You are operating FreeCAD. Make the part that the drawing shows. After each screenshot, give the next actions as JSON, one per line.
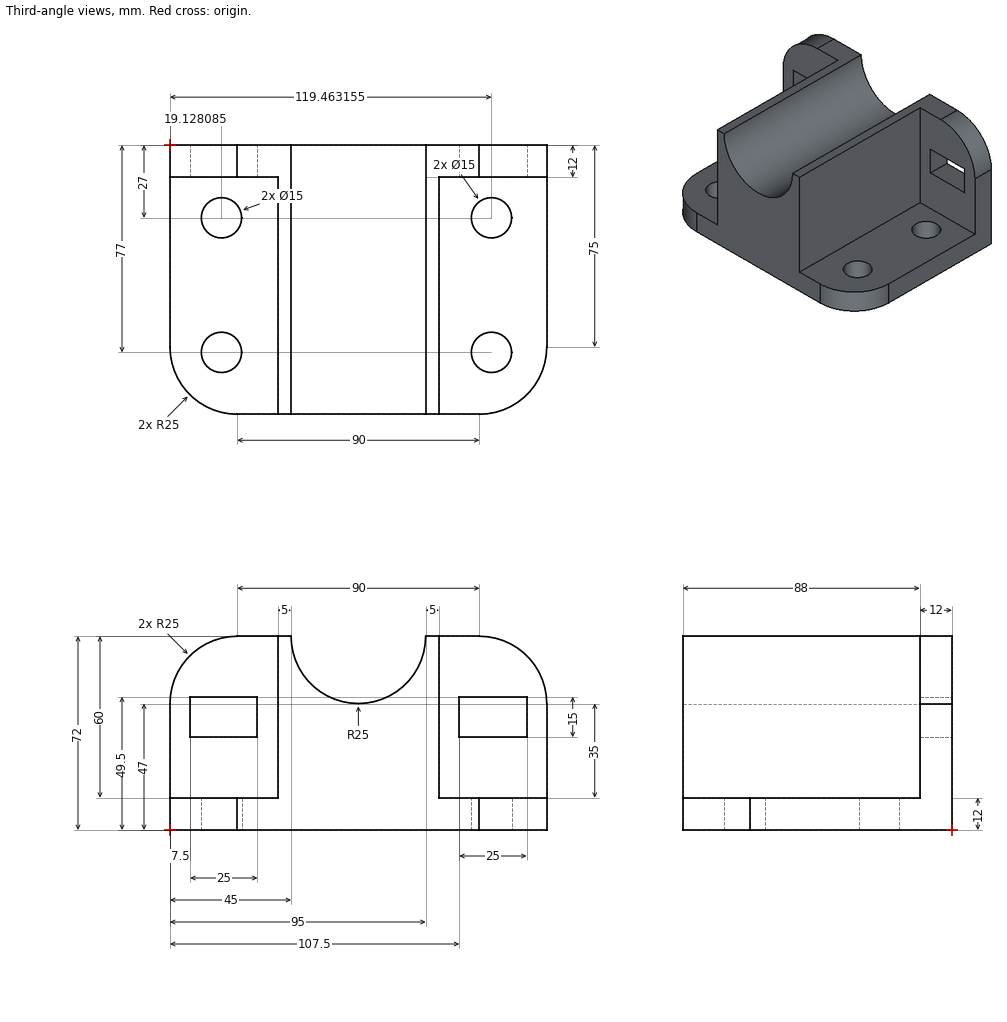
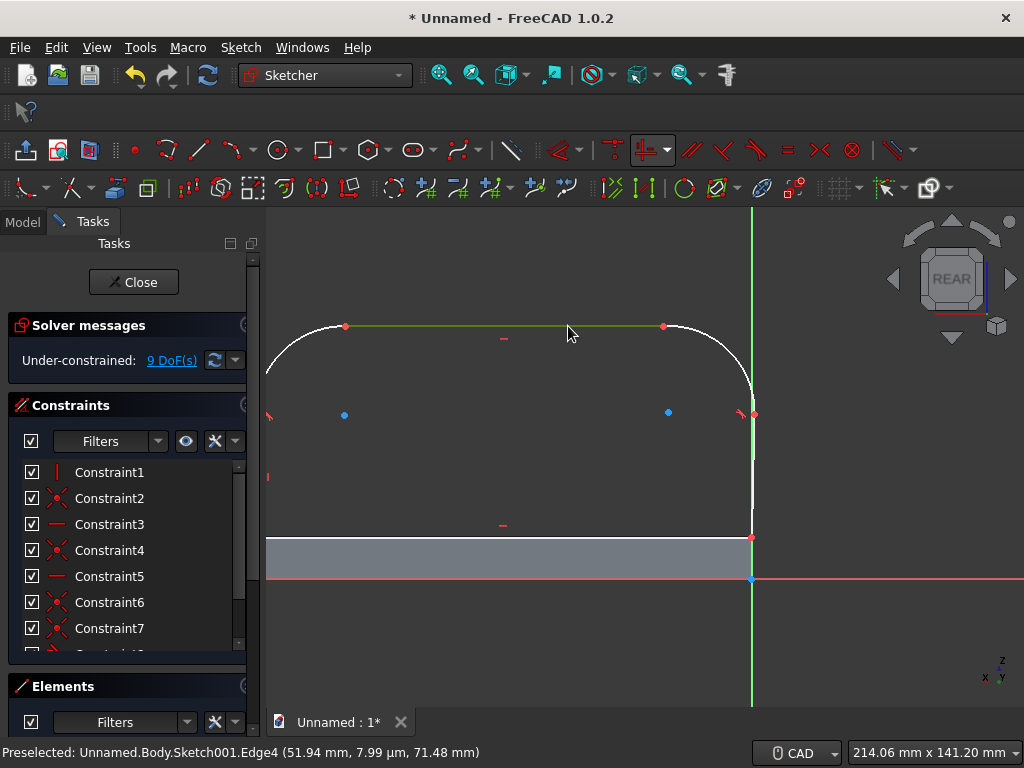
{"action": "left_click", "coordinate": [705, 334]}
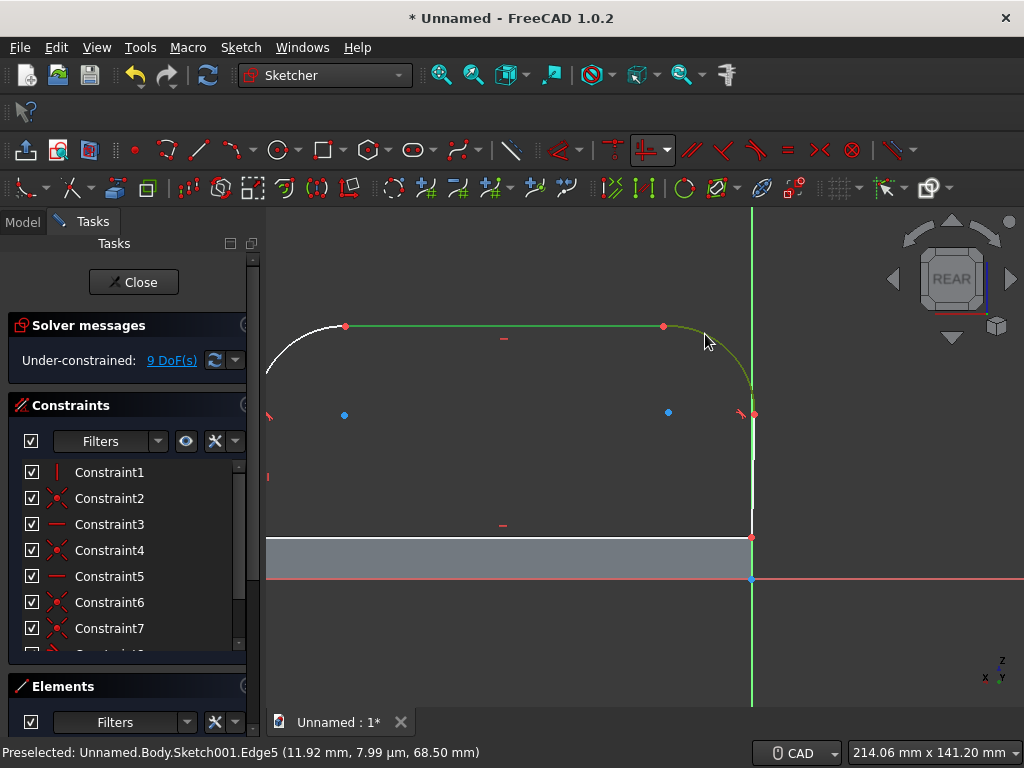
{"action": "key", "text": "t"}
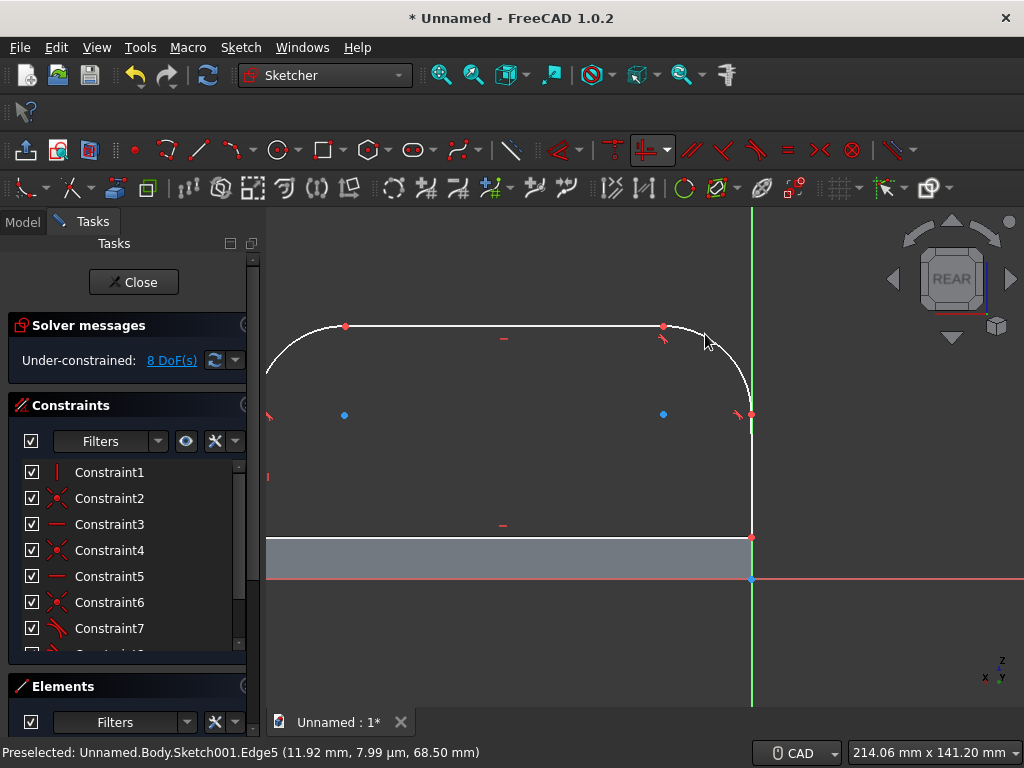
{"action": "left_click", "coordinate": [568, 326]}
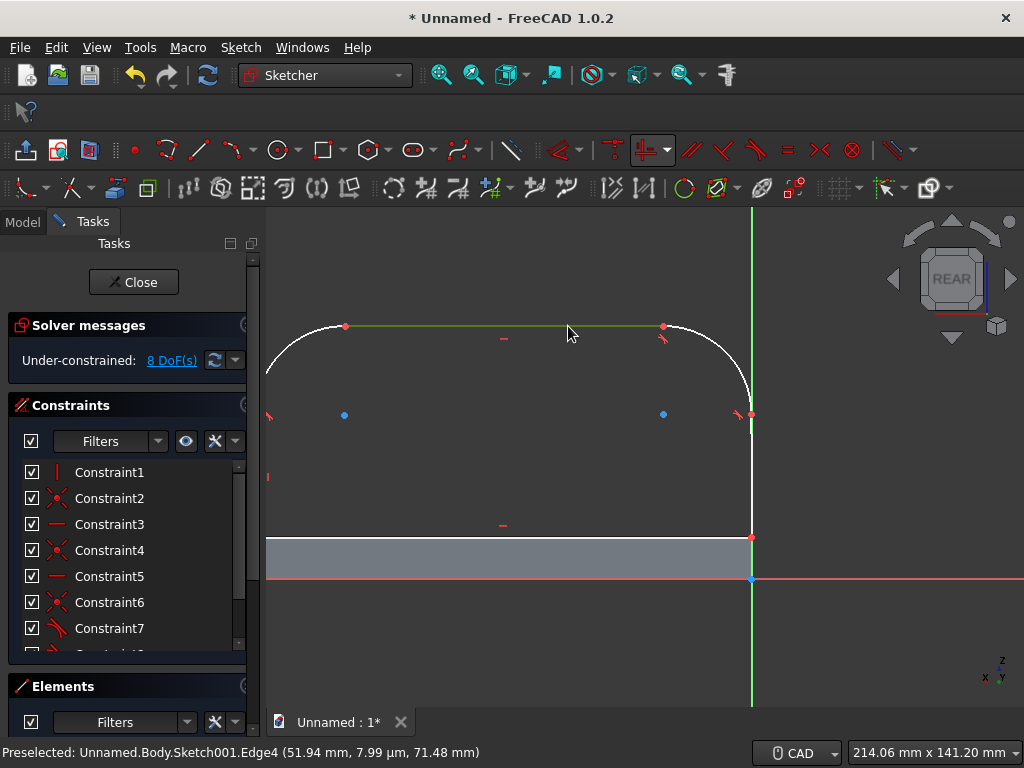
{"action": "left_click", "coordinate": [305, 336]}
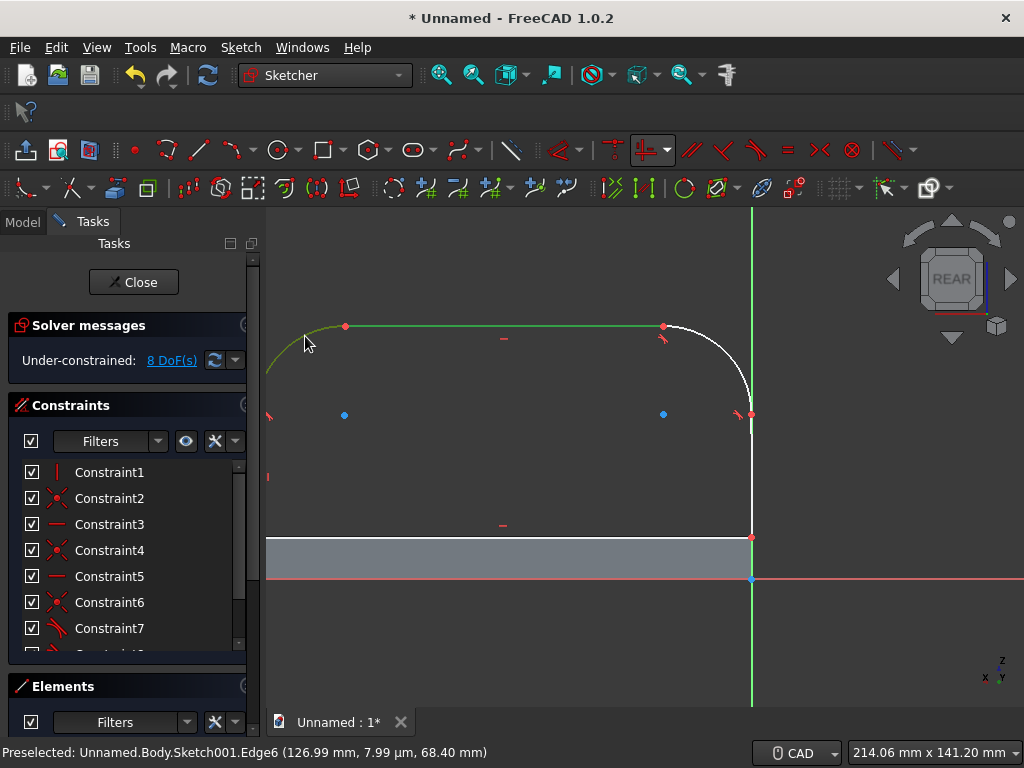
{"action": "key", "text": "t"}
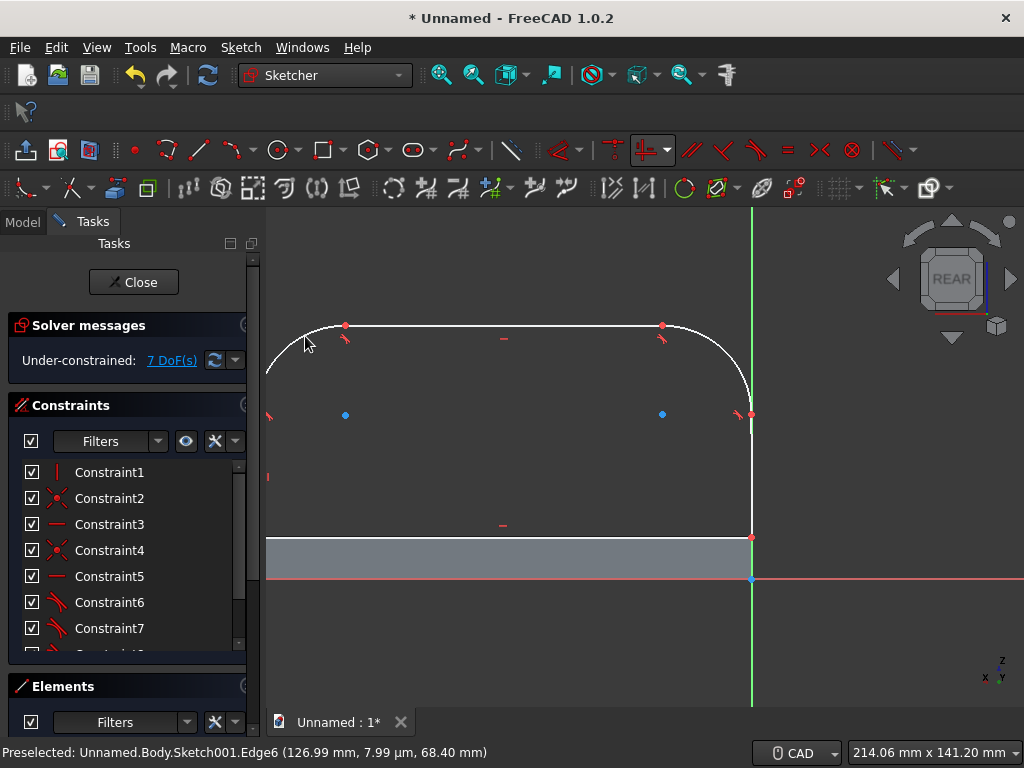
{"action": "left_click", "coordinate": [752, 501]}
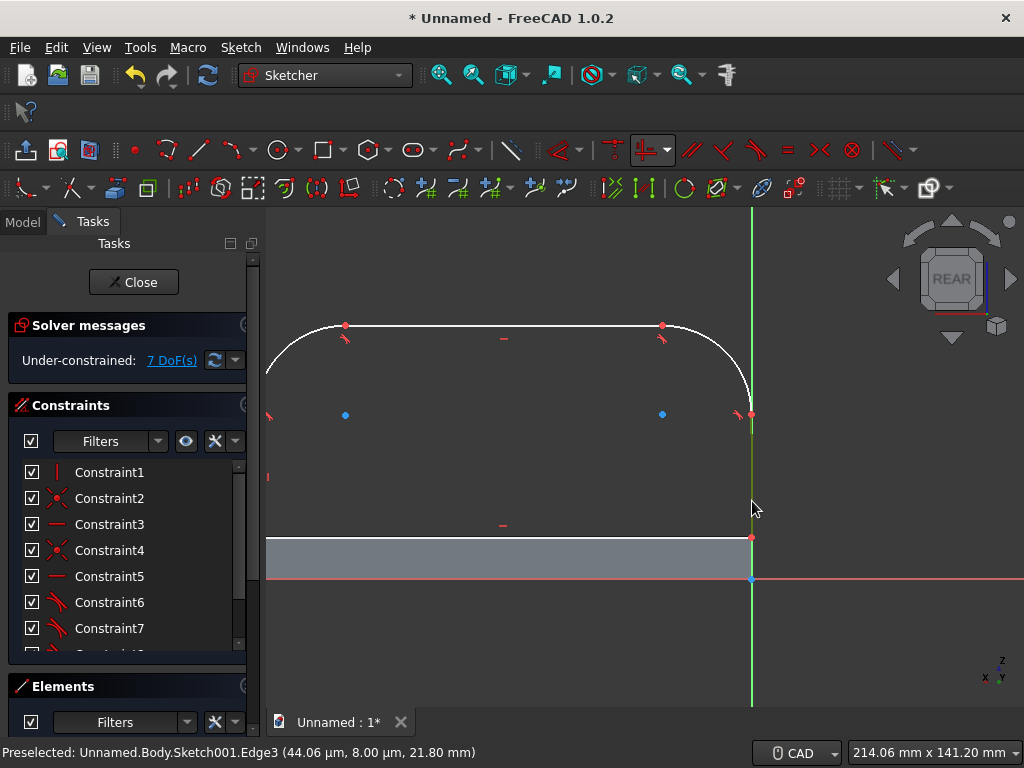
{"action": "key", "text": "v"}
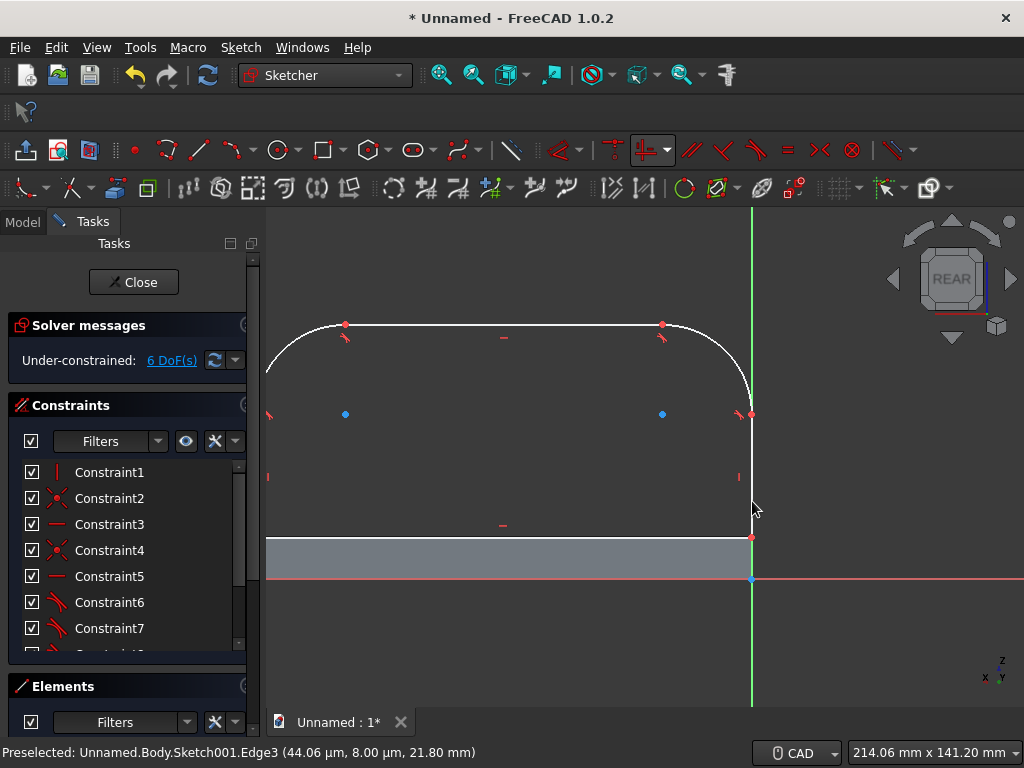
{"action": "scroll", "coordinate": [742, 374], "scroll_direction": "up", "scroll_amount": 2}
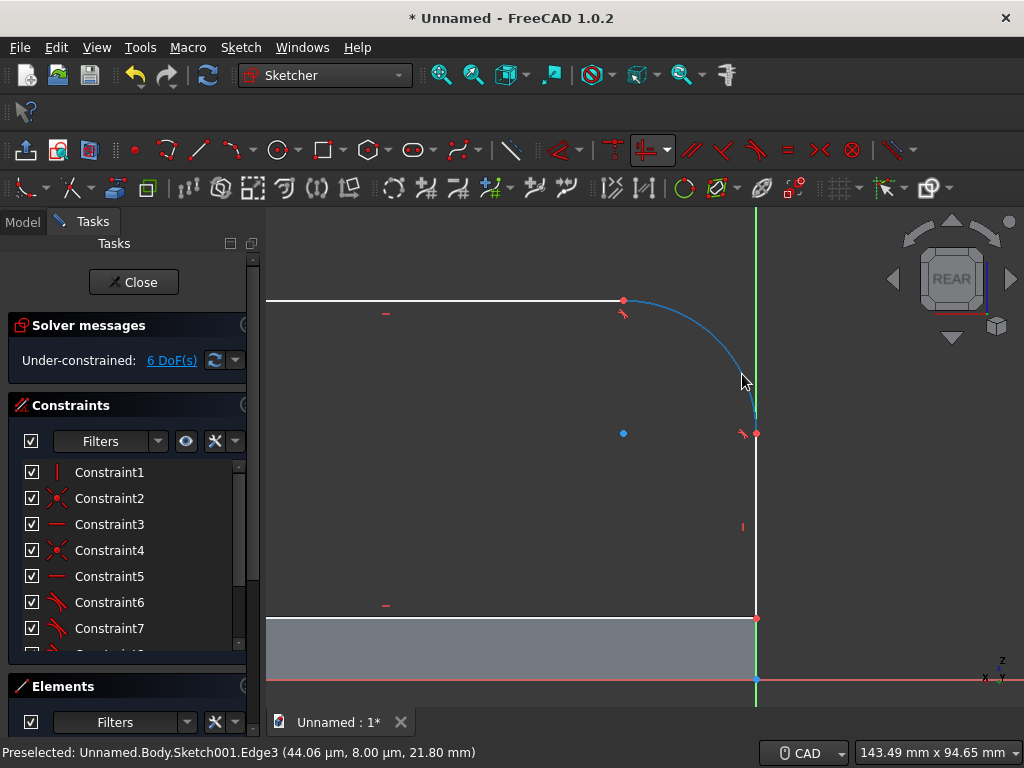
{"action": "left_click", "coordinate": [742, 373]}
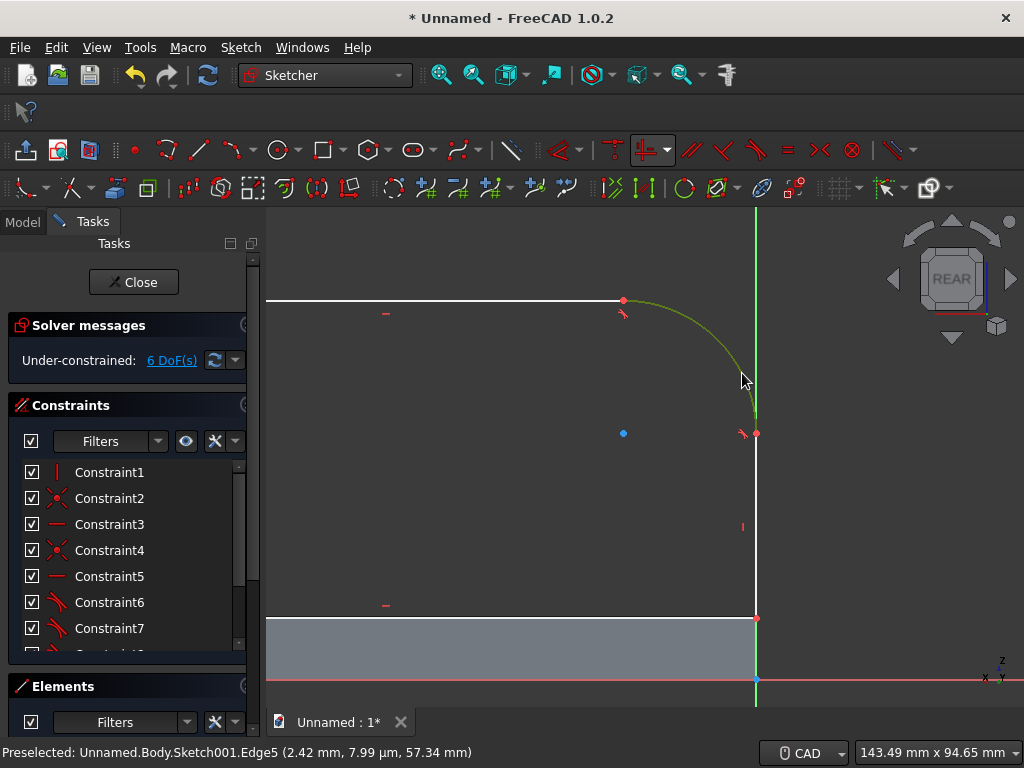
{"action": "scroll", "coordinate": [807, 417], "scroll_direction": "down", "scroll_amount": 3}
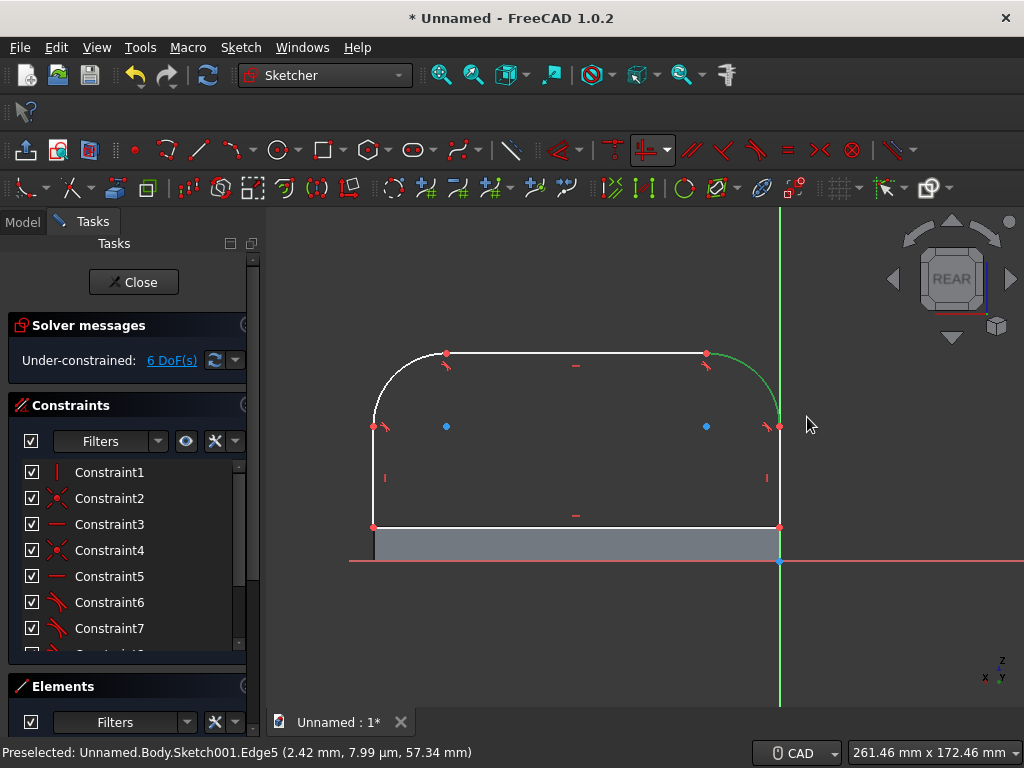
{"action": "left_click", "coordinate": [413, 361]}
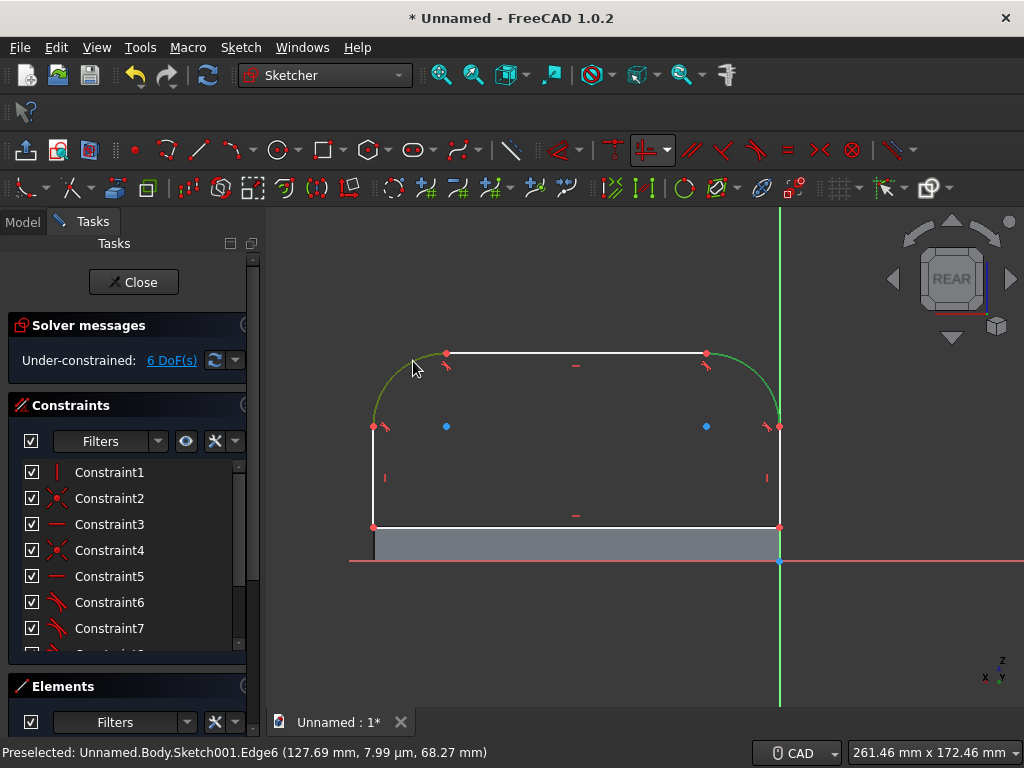
{"action": "left_click", "coordinate": [788, 150]}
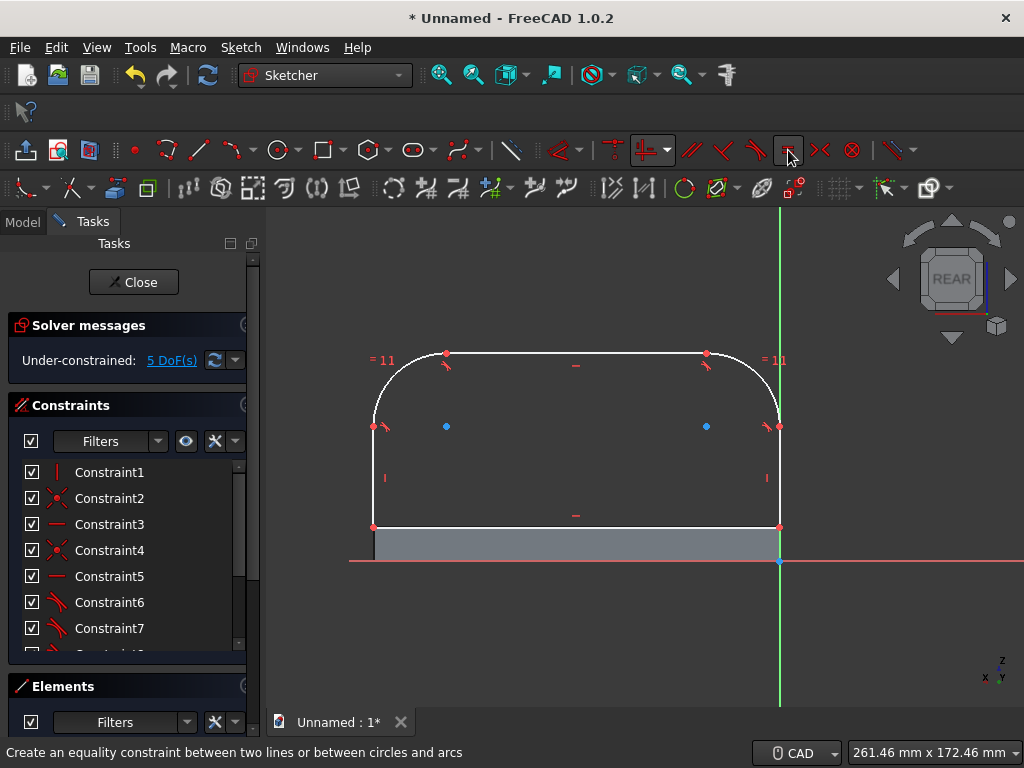
{"action": "left_click", "coordinate": [740, 361]}